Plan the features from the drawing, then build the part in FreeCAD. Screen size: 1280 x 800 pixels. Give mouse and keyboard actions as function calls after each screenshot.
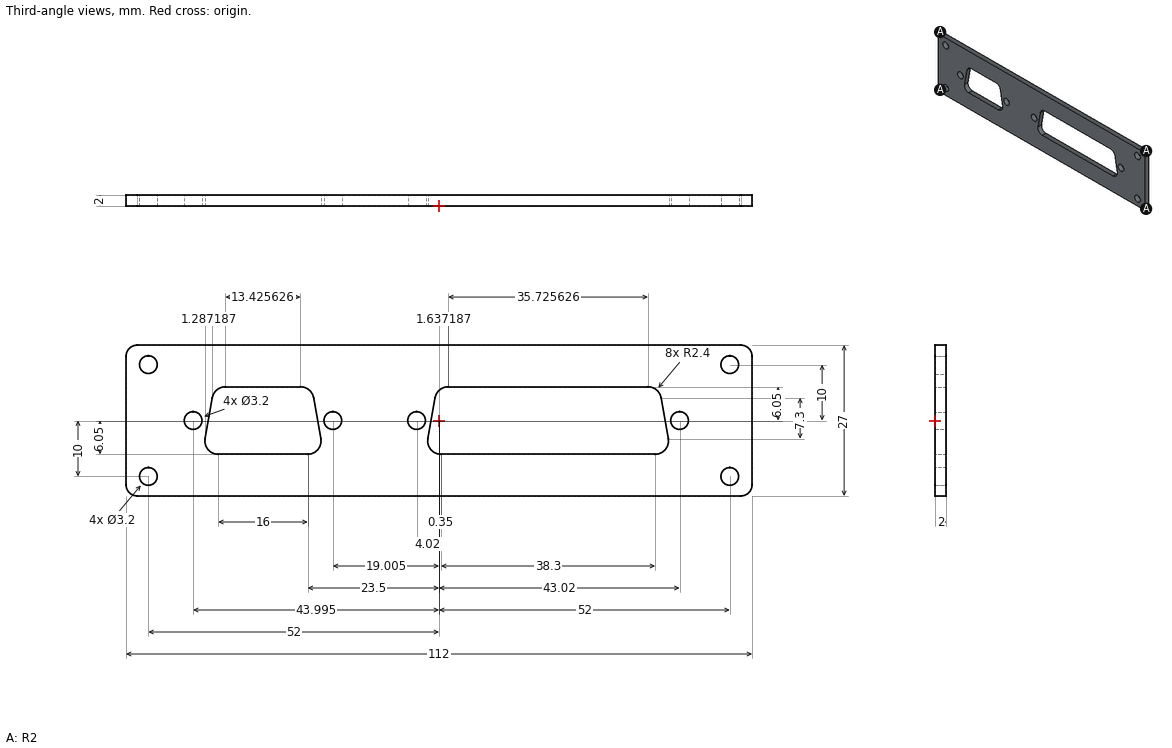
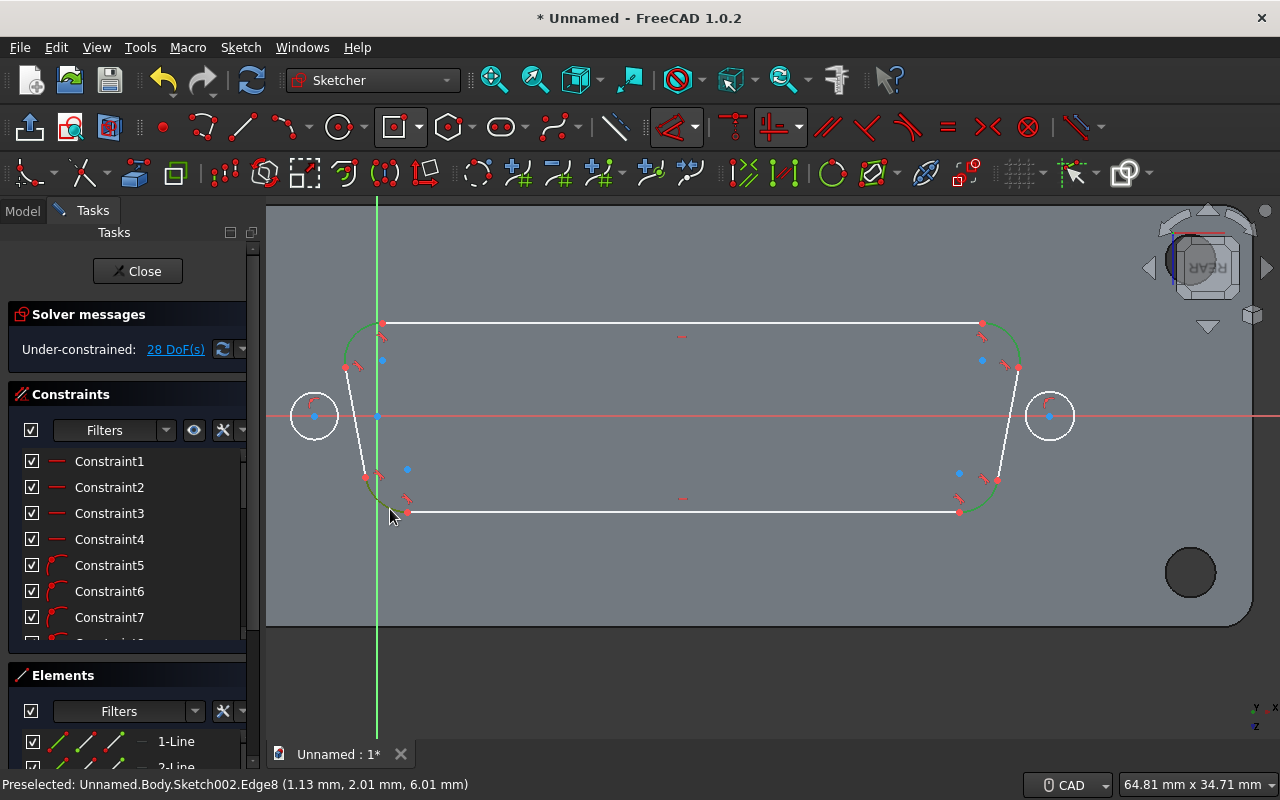
scroll(978, 509, down, 4)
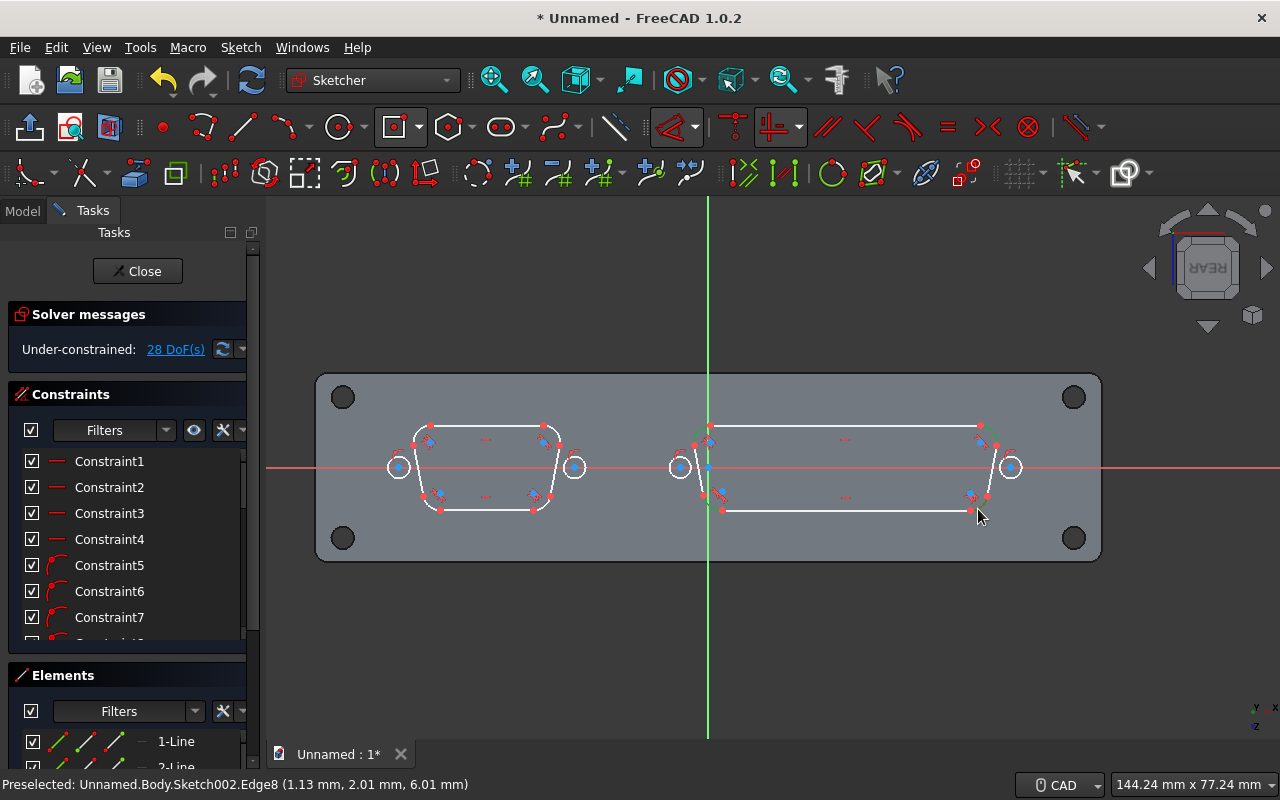
scroll(422, 428, up, 3)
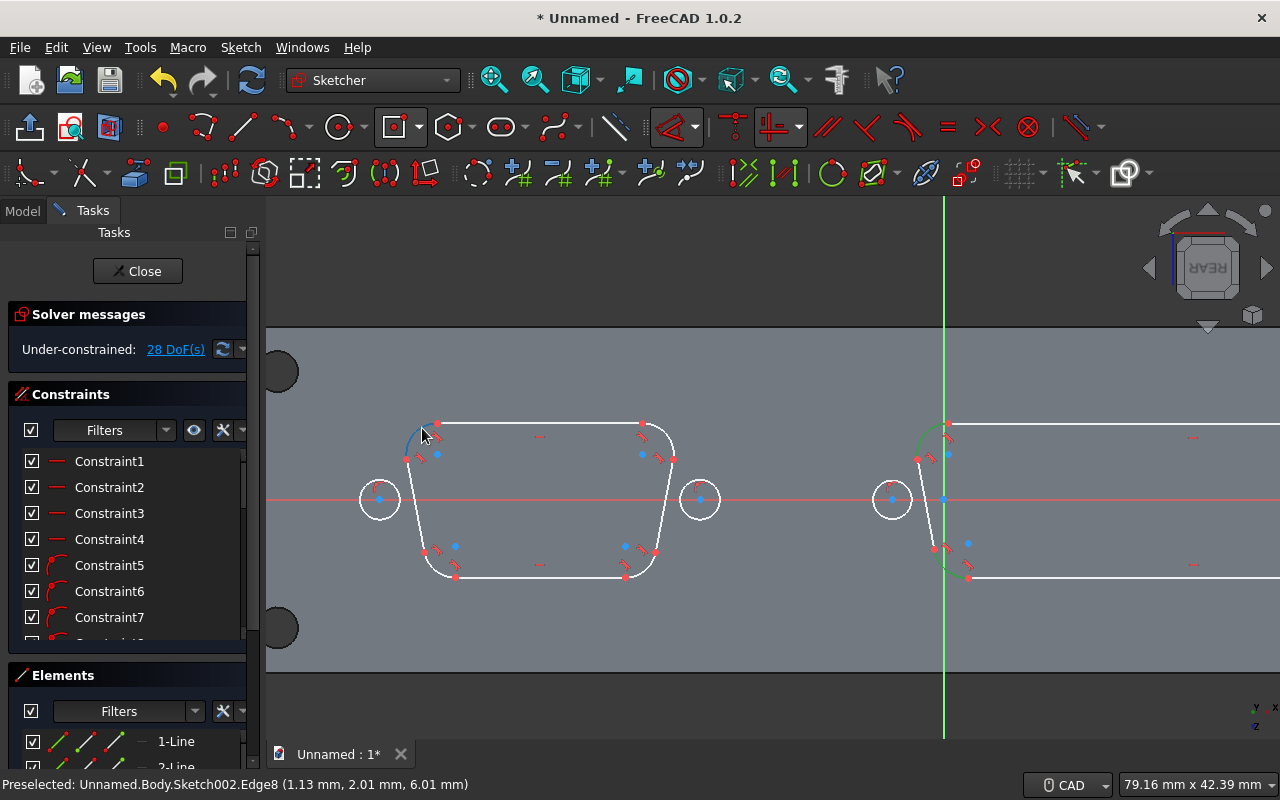
click(422, 428)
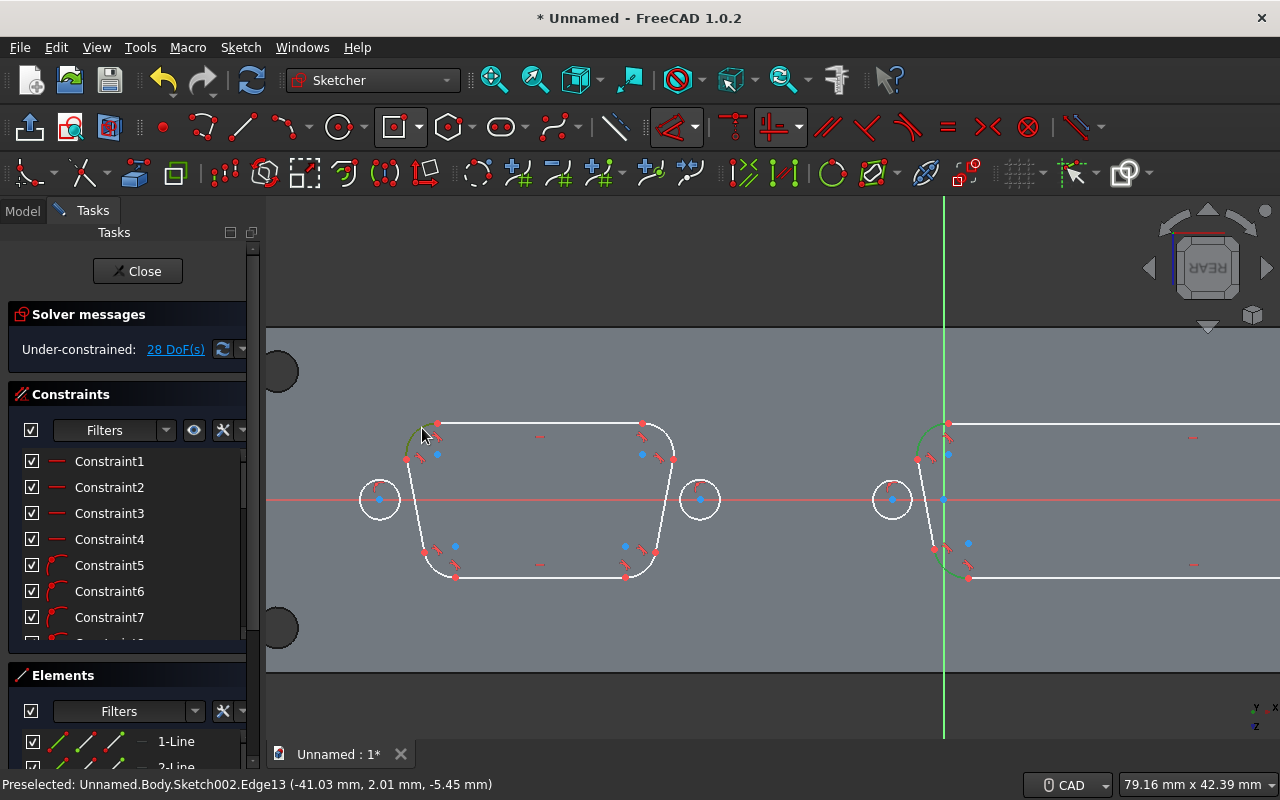
click(430, 564)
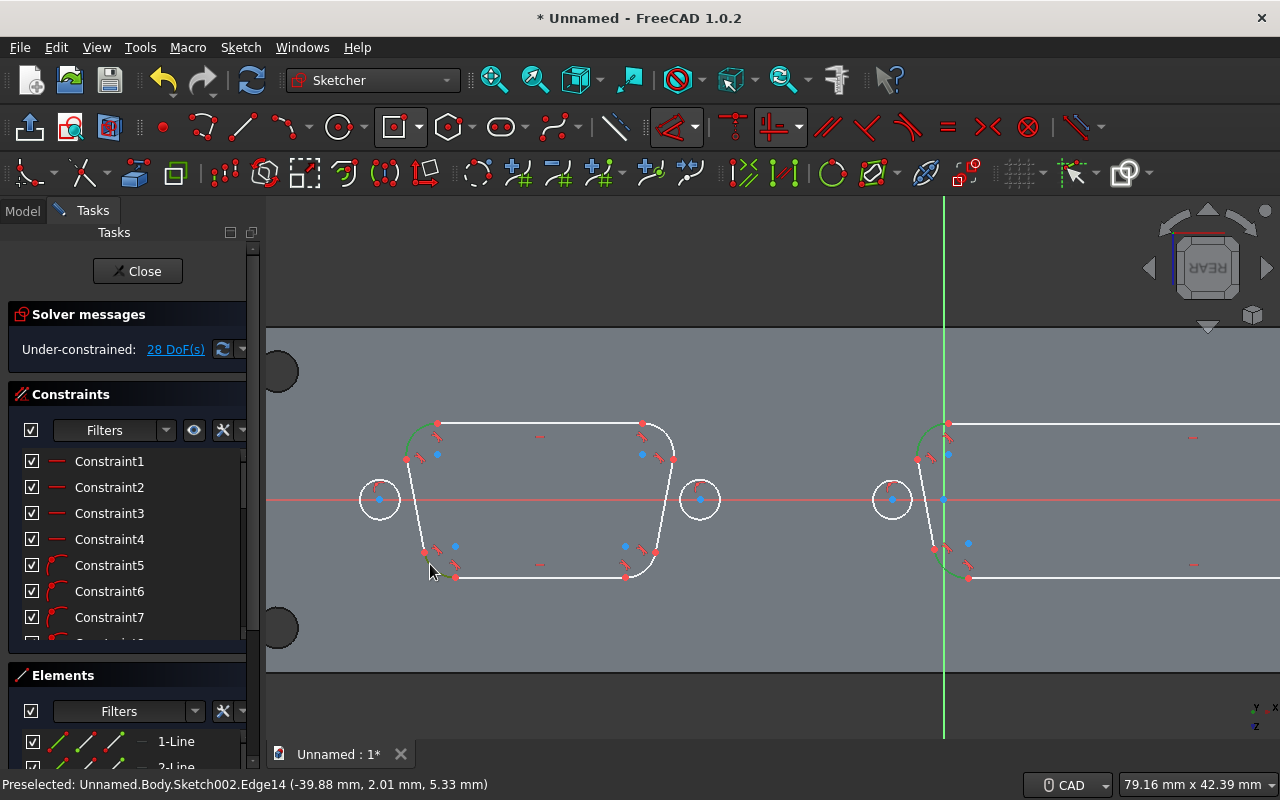
click(638, 575)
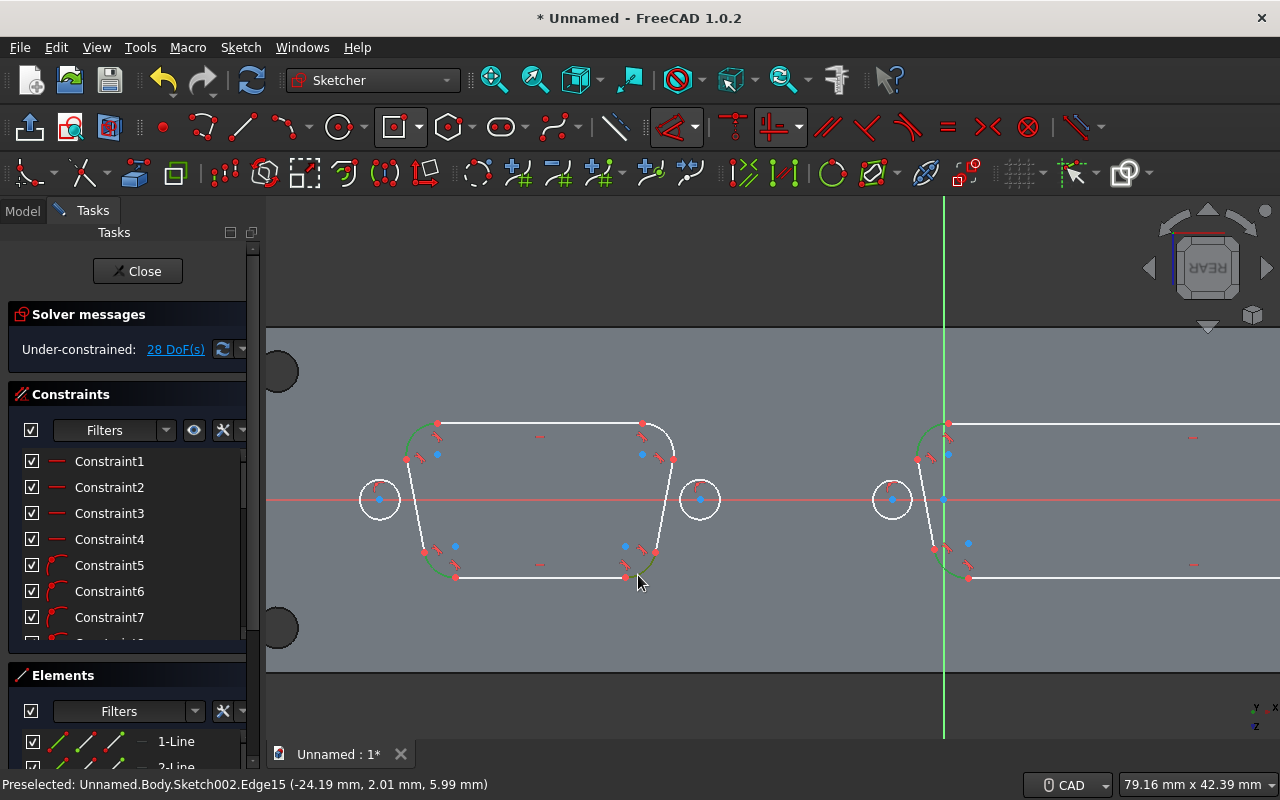
click(672, 444)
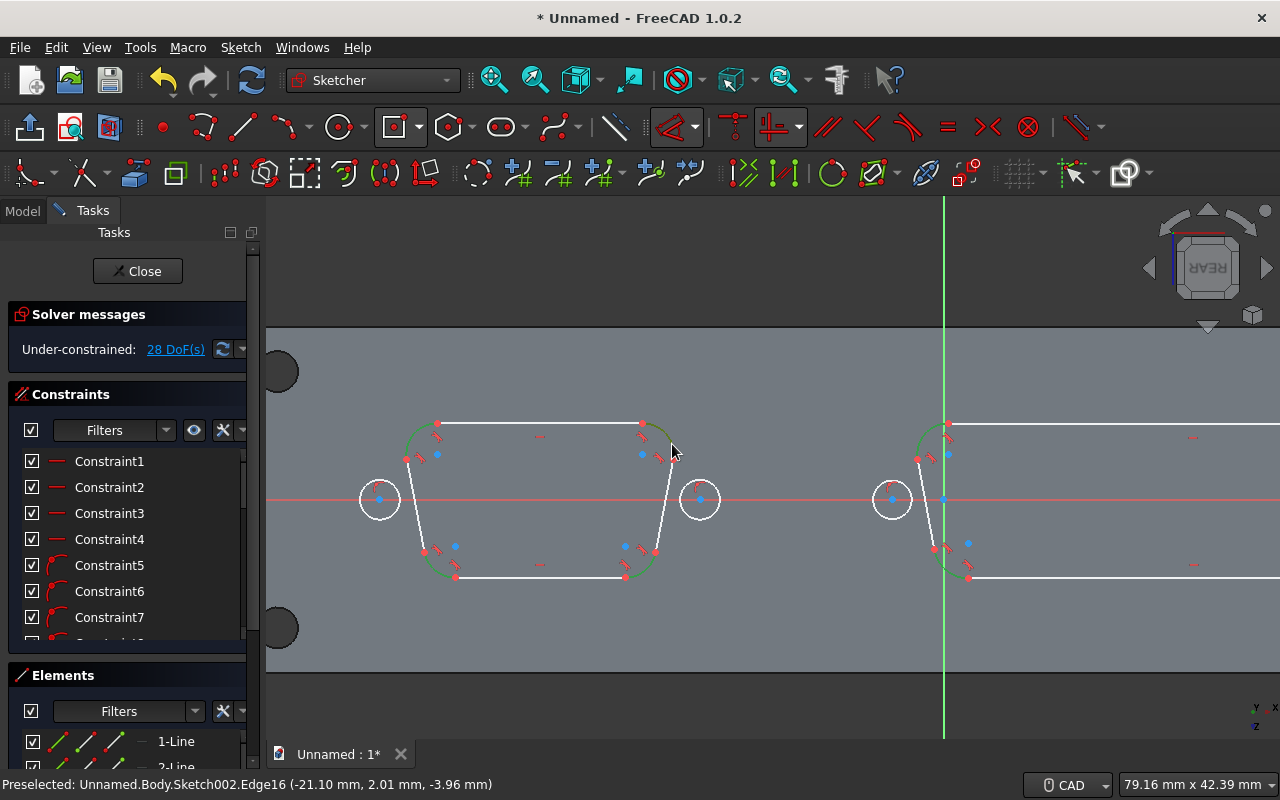
key(e)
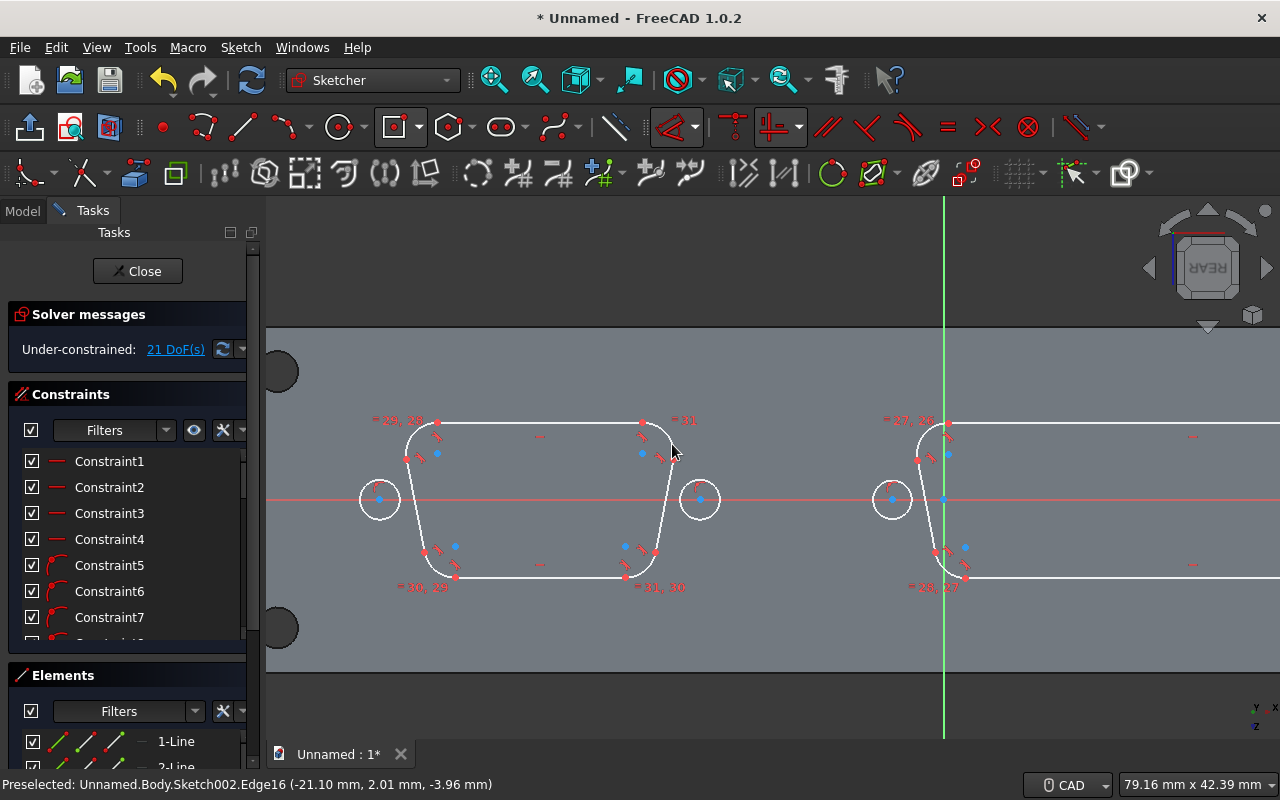
click(394, 486)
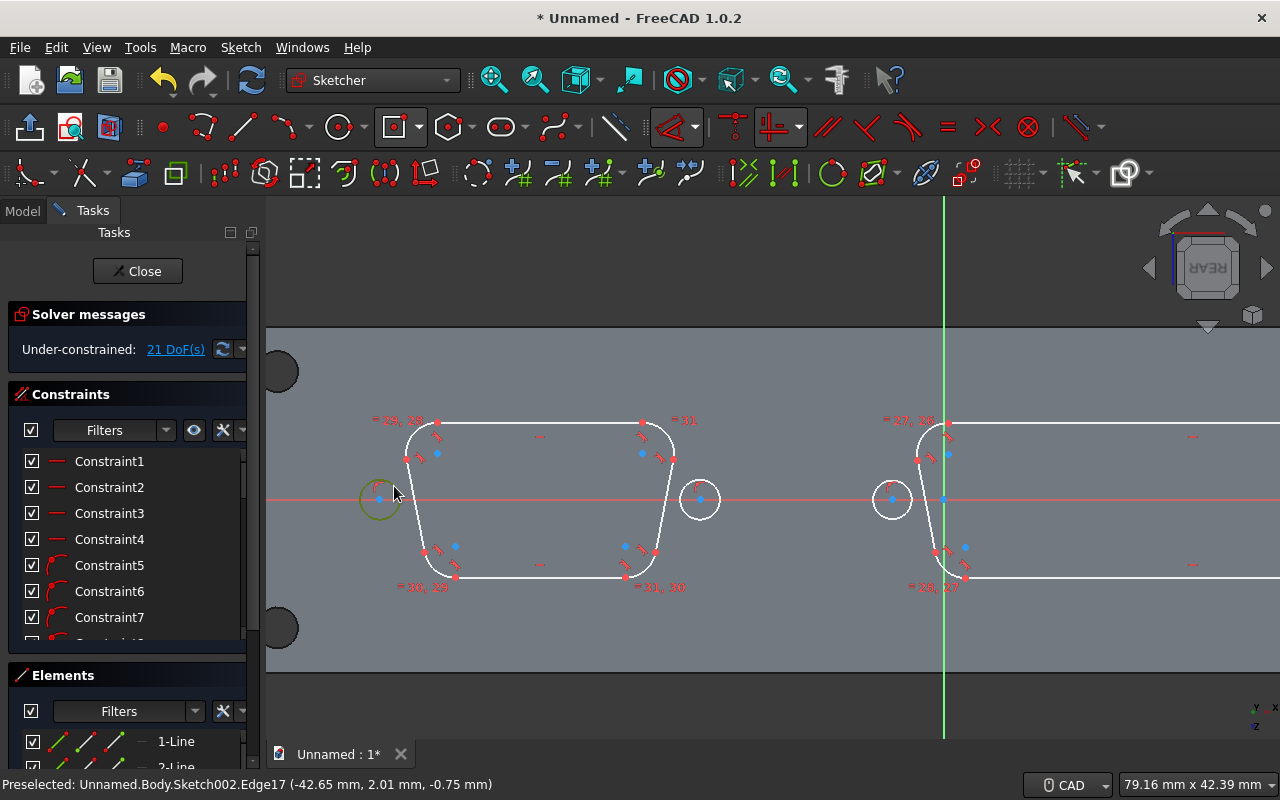
click(714, 486)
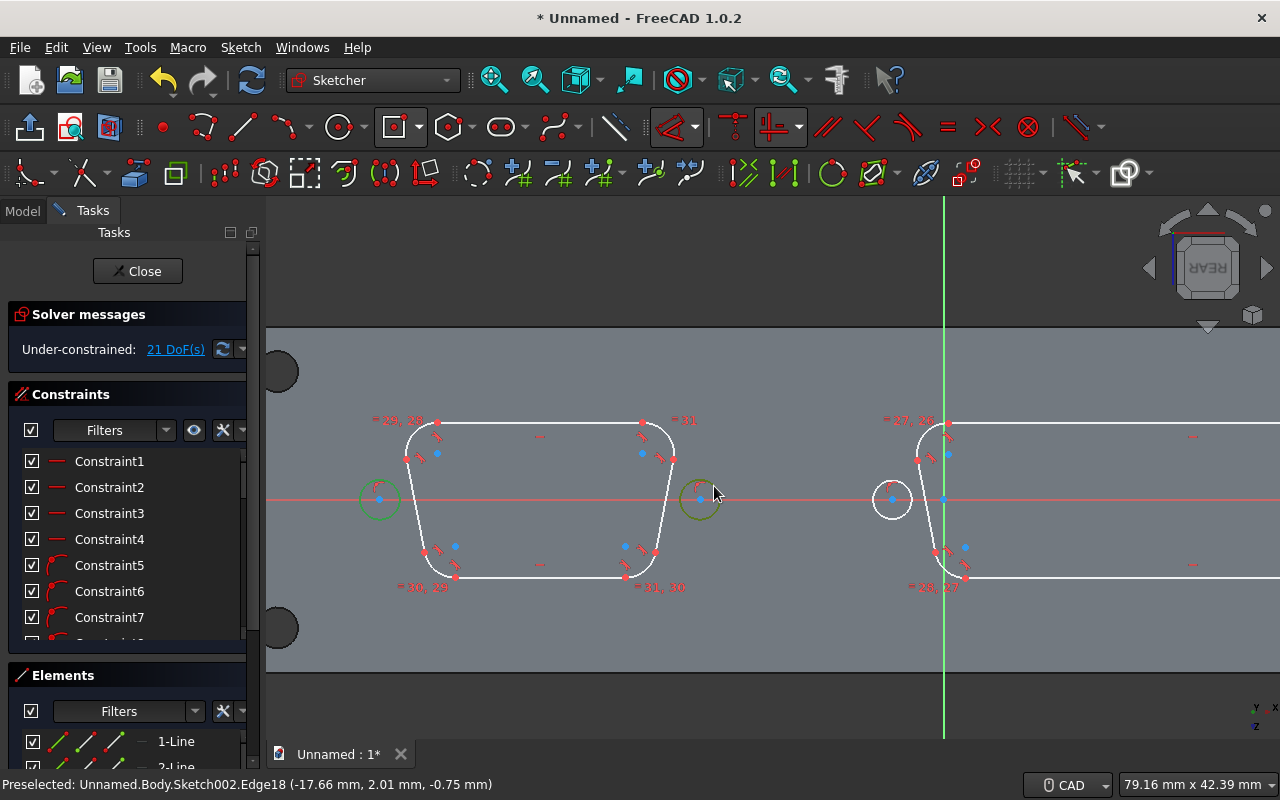
click(906, 486)